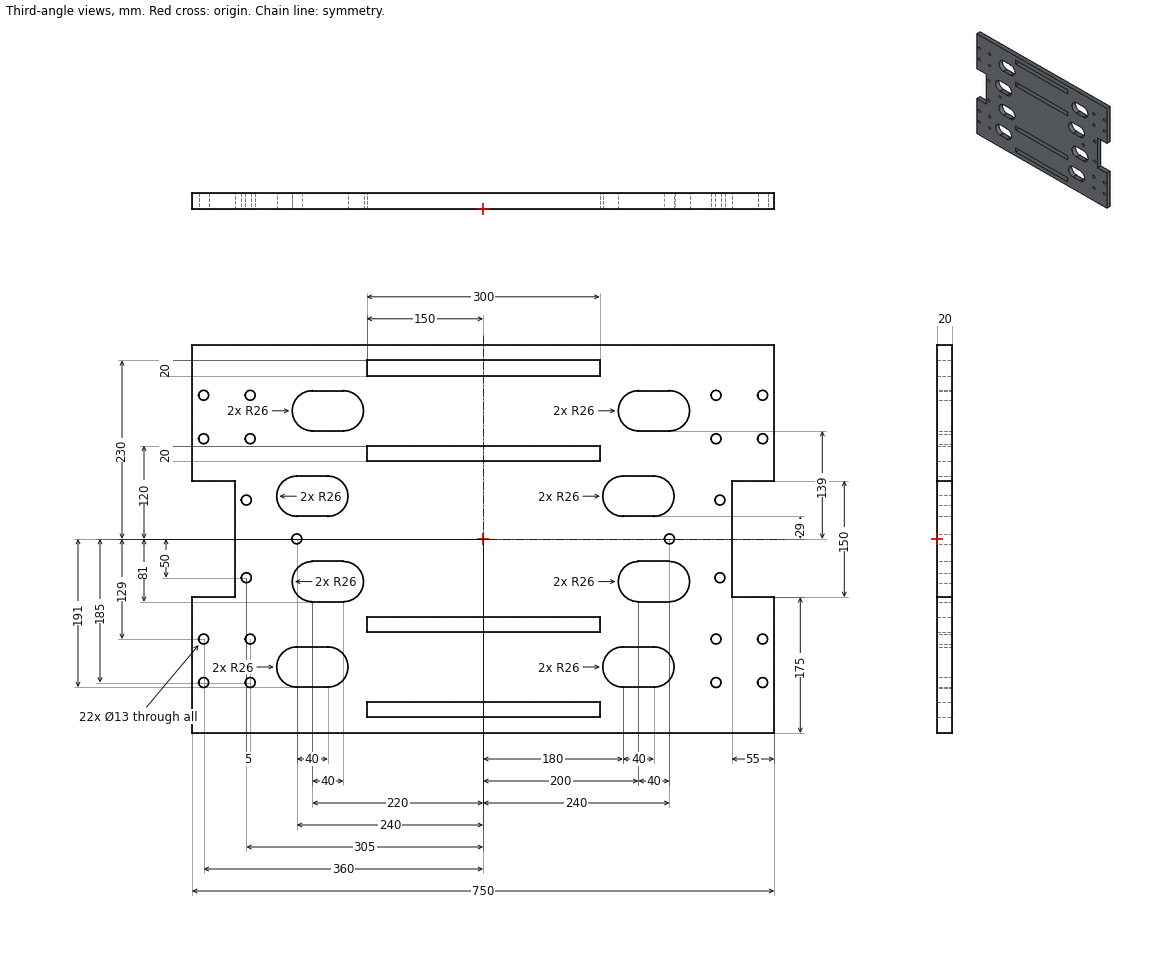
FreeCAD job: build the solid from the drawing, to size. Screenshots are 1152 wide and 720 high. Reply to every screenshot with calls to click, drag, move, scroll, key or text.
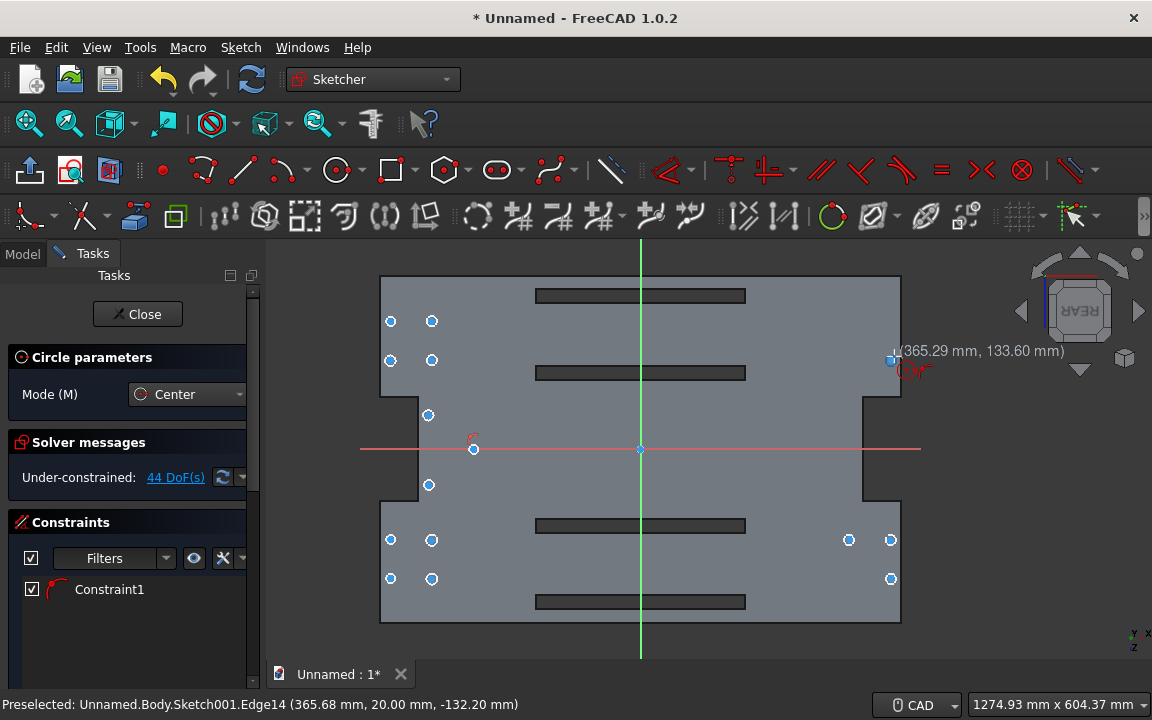
scroll(891, 321, up, 9)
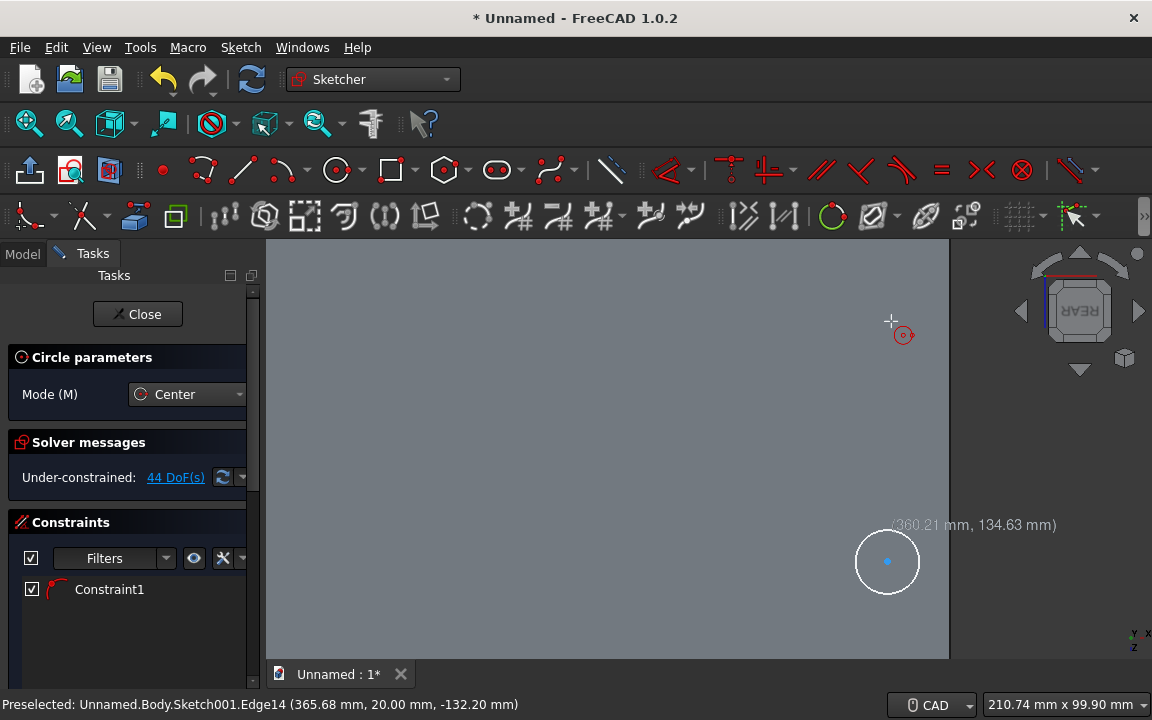
scroll(891, 321, down, 9)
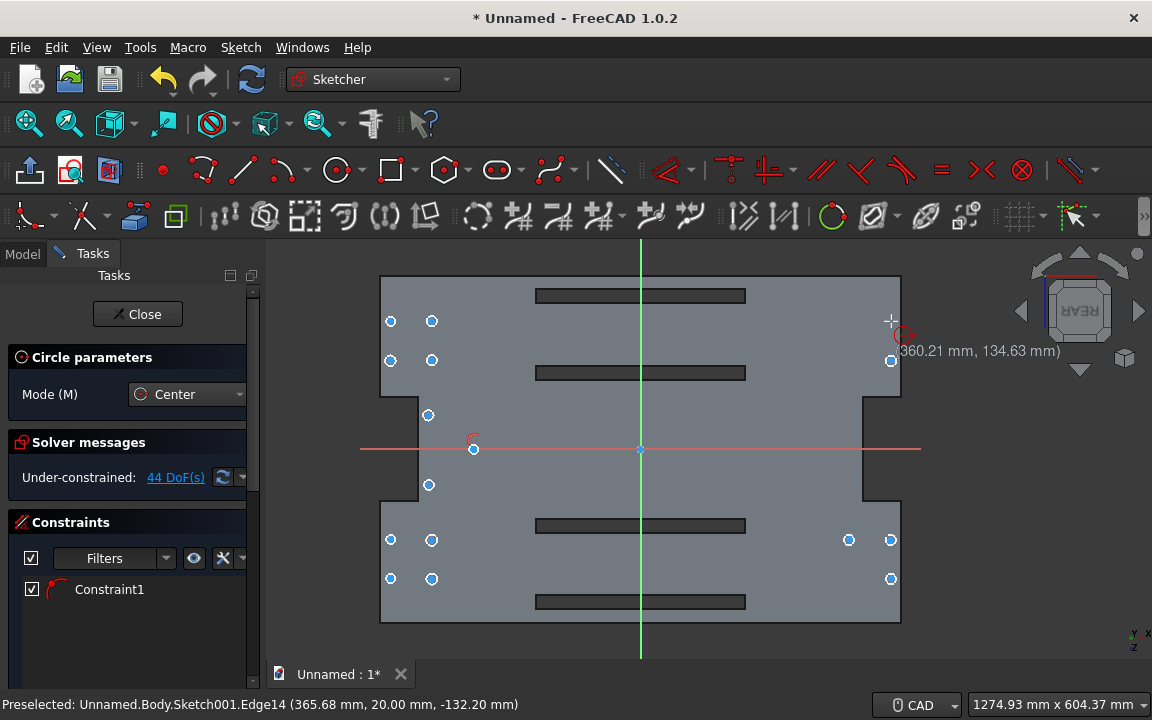
click(891, 321)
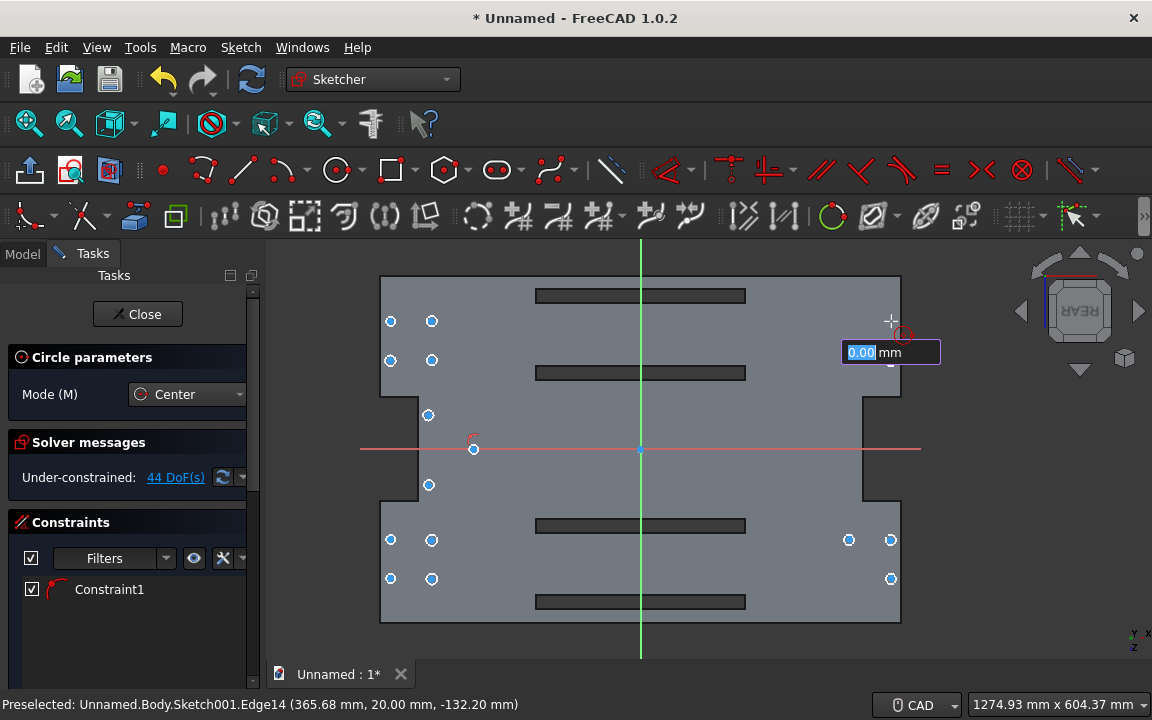
scroll(894, 318, up, 7)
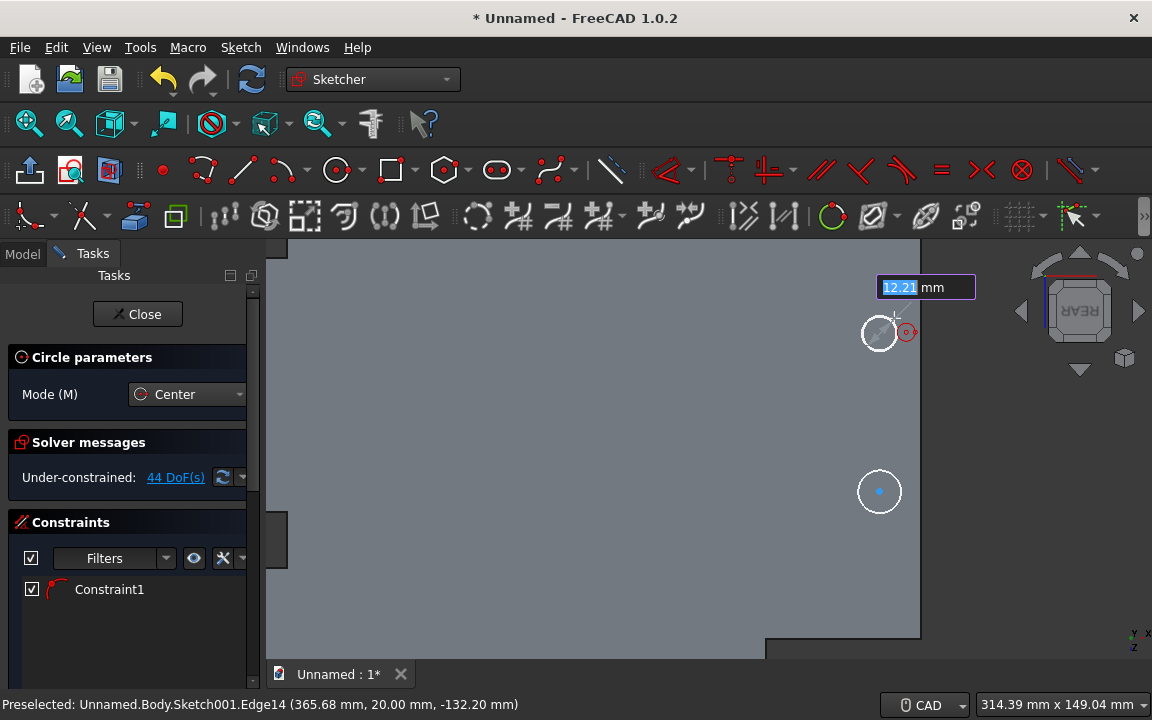
click(892, 316)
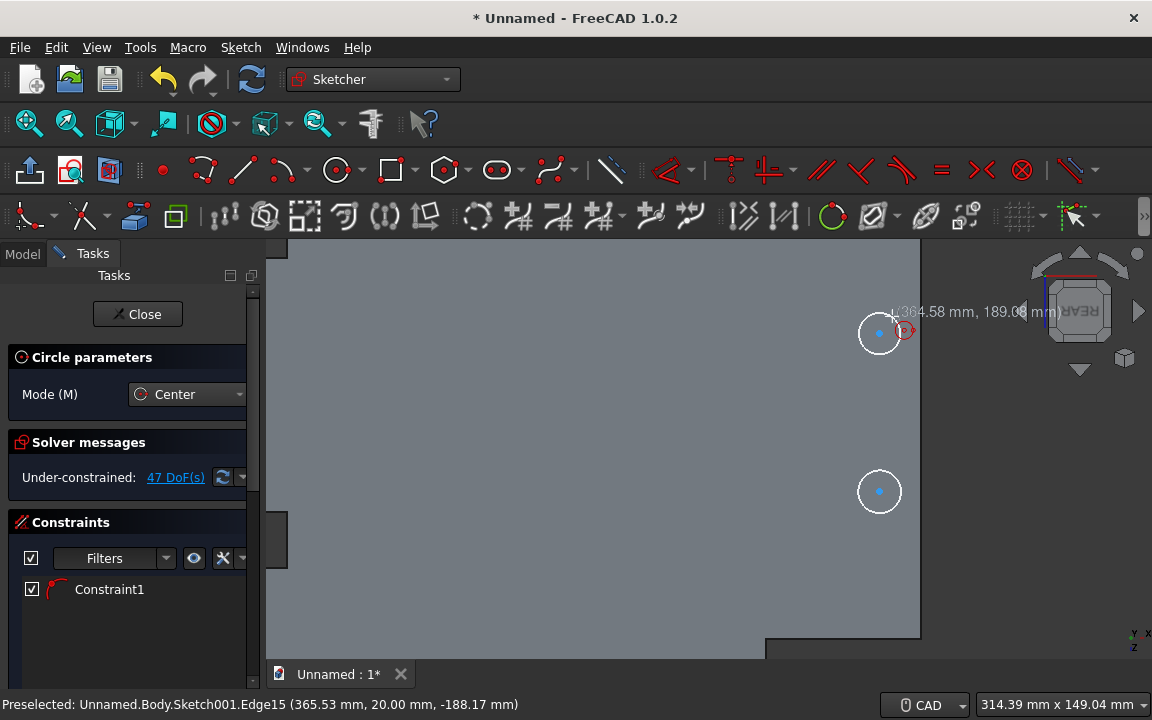
scroll(710, 486, up, 2)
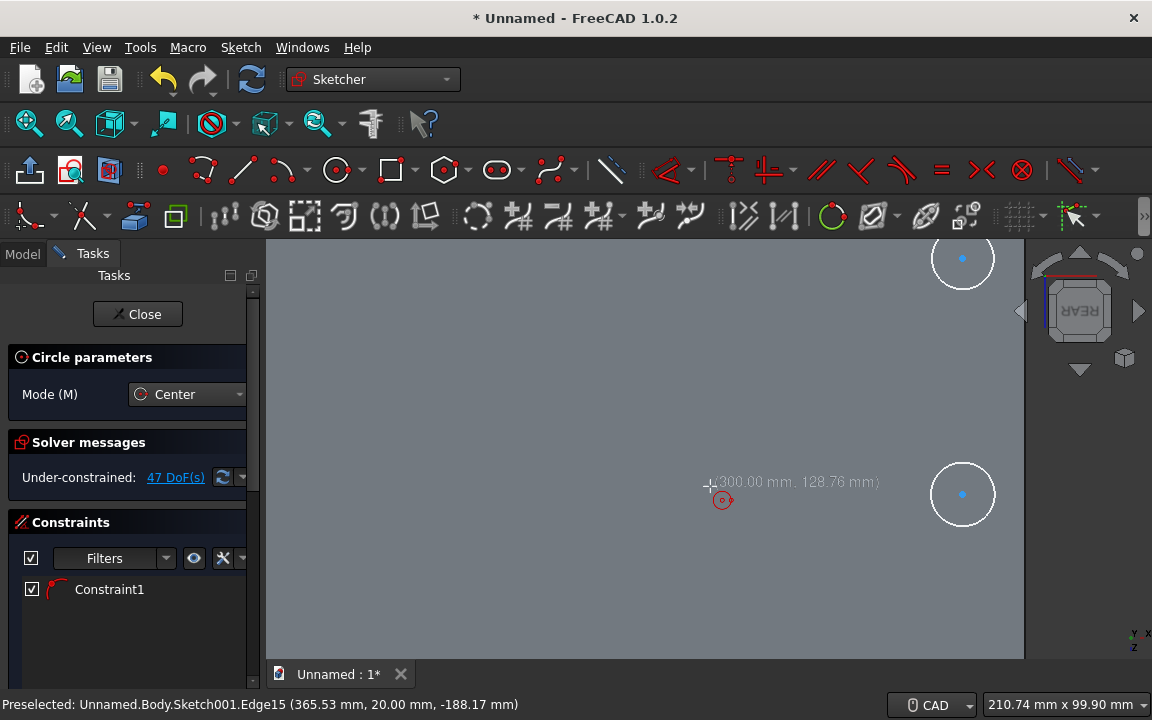
scroll(877, 334, down, 9)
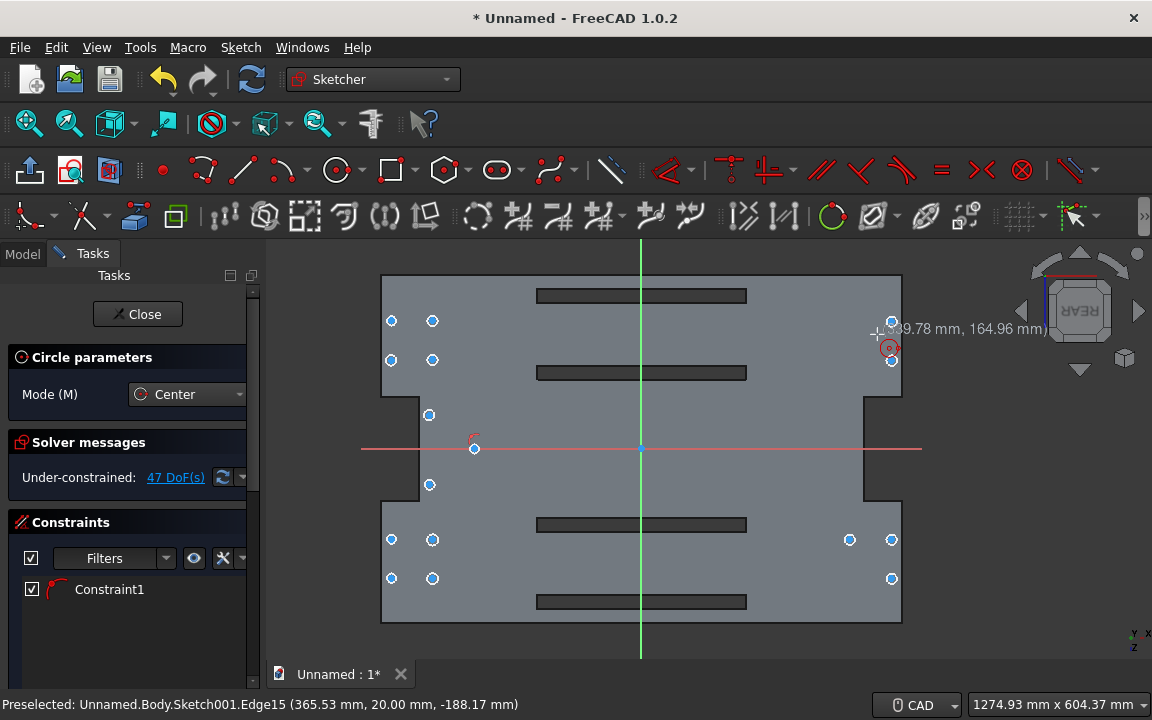
click(850, 359)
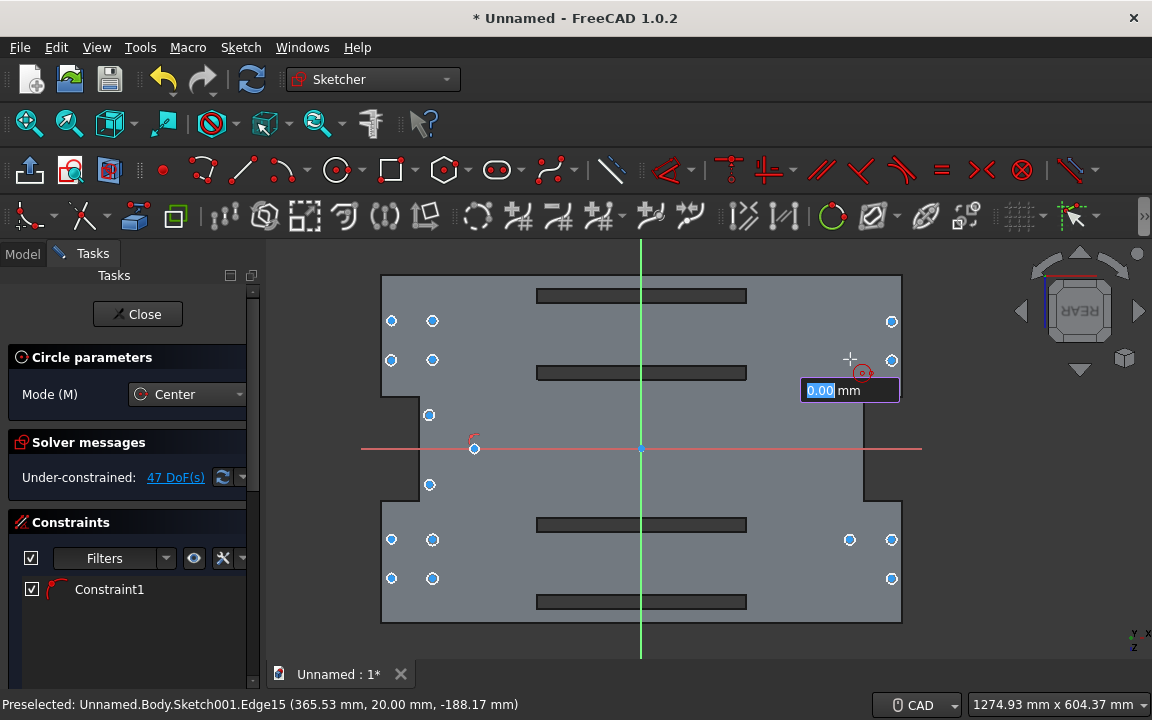
scroll(853, 356, up, 7)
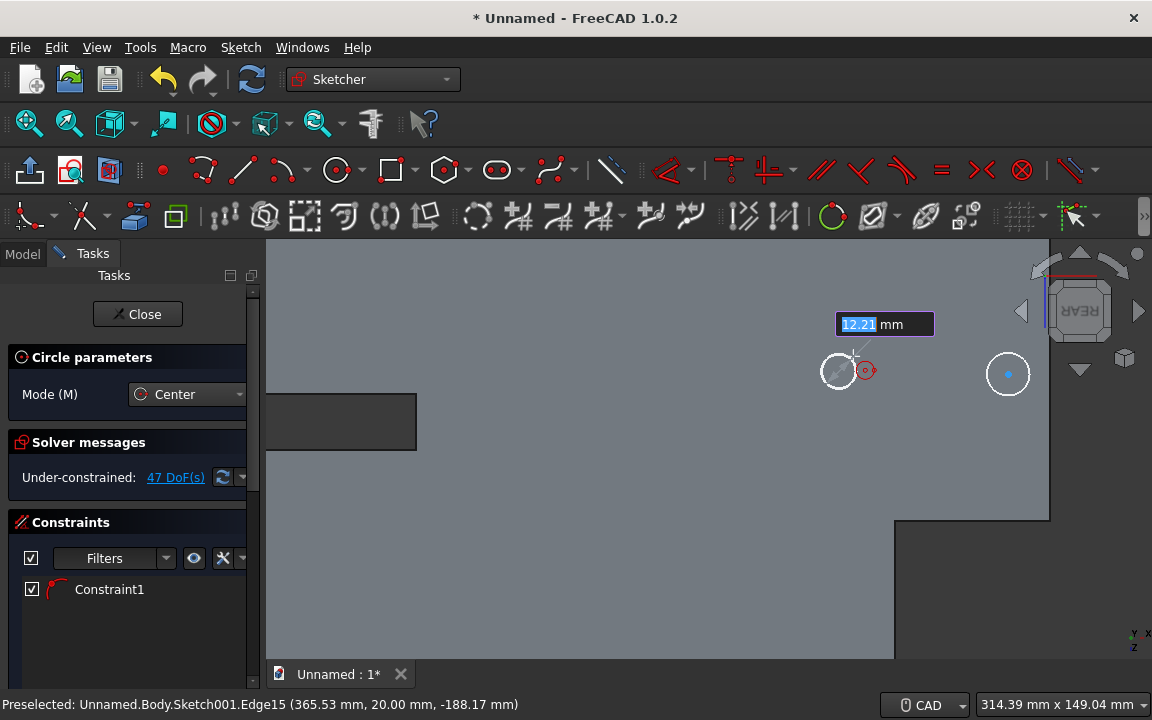
click(851, 356)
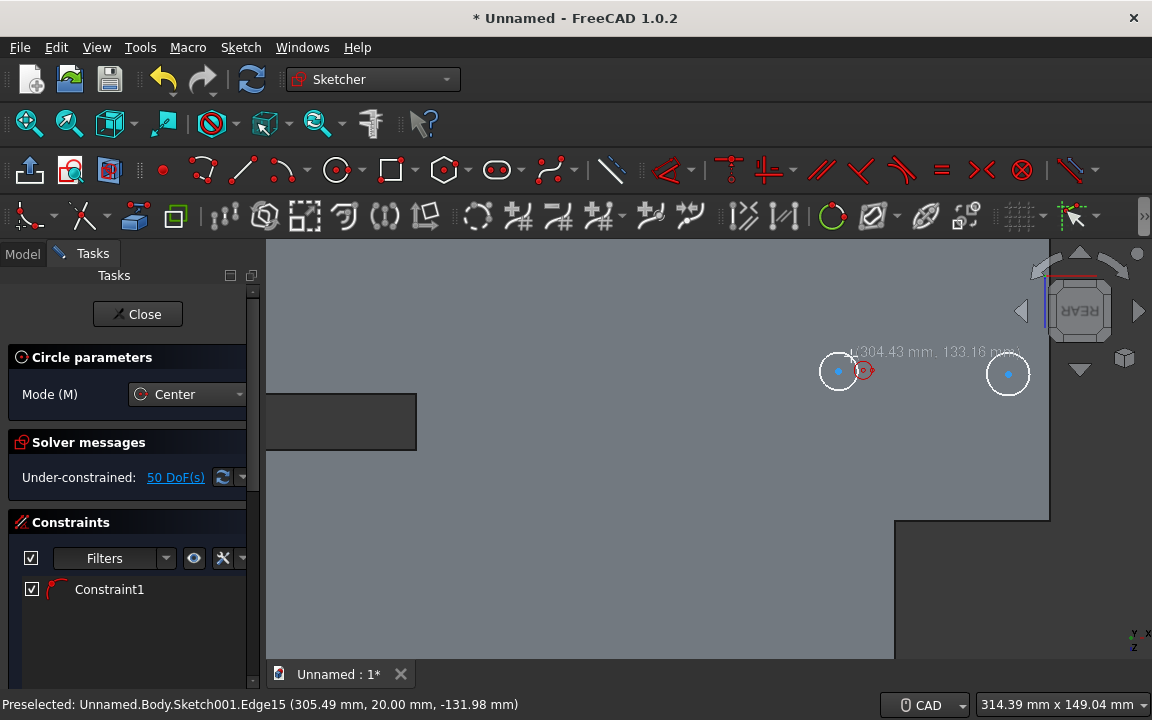
scroll(852, 356, down, 7)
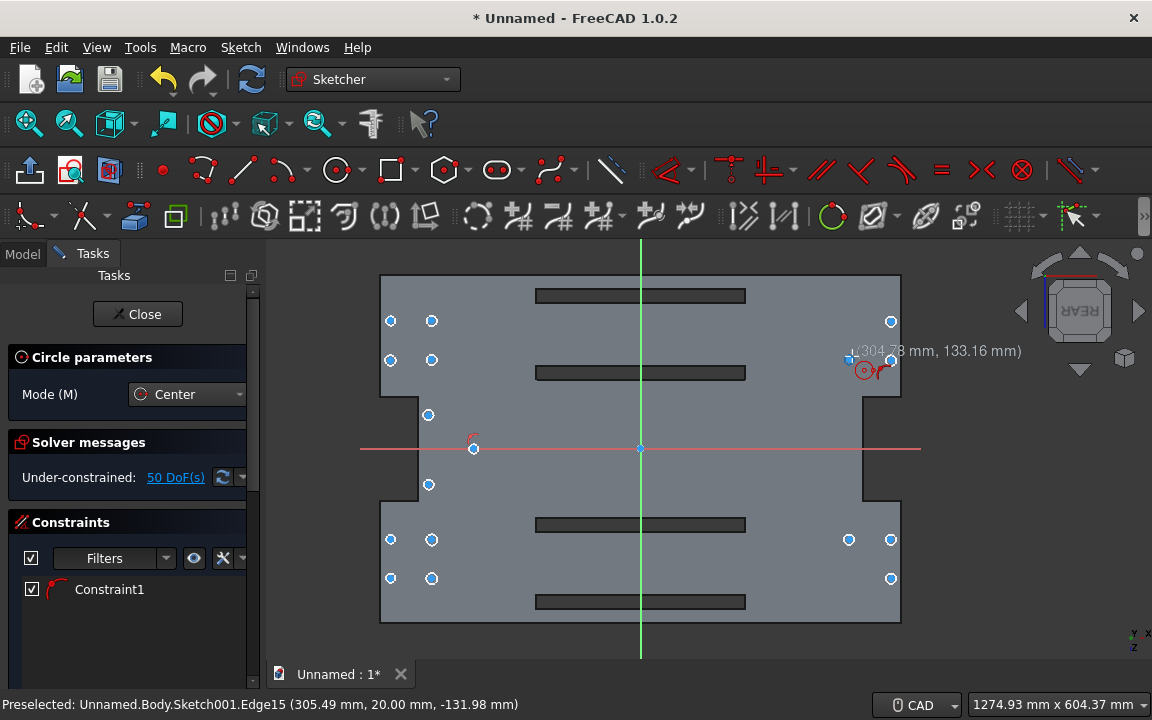
scroll(853, 484, up, 9)